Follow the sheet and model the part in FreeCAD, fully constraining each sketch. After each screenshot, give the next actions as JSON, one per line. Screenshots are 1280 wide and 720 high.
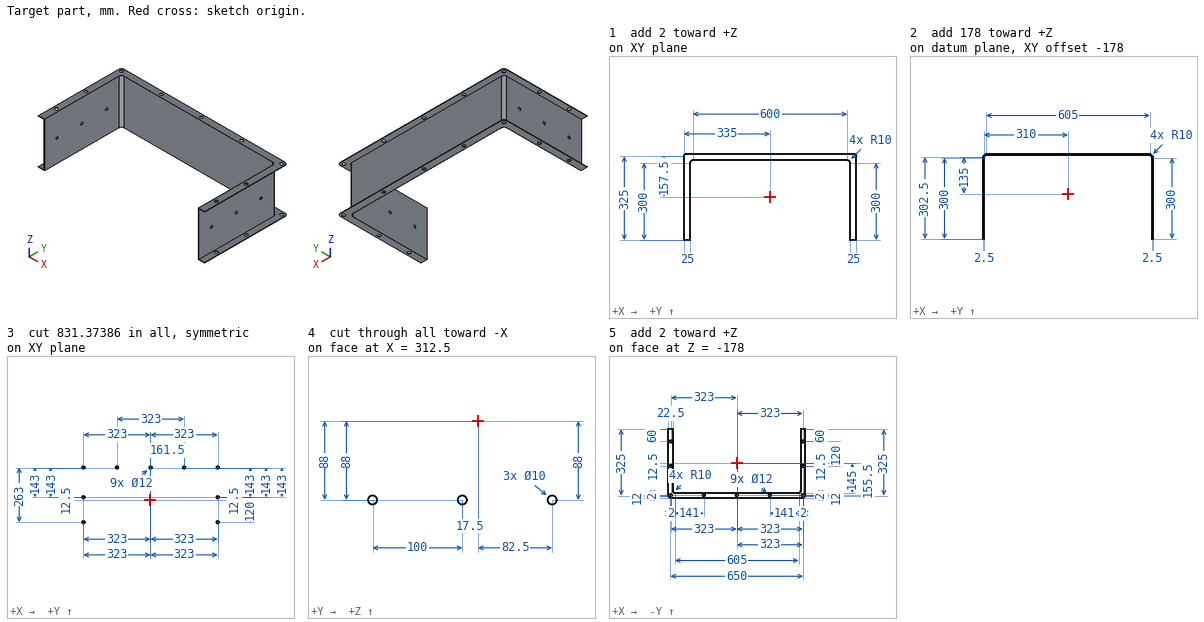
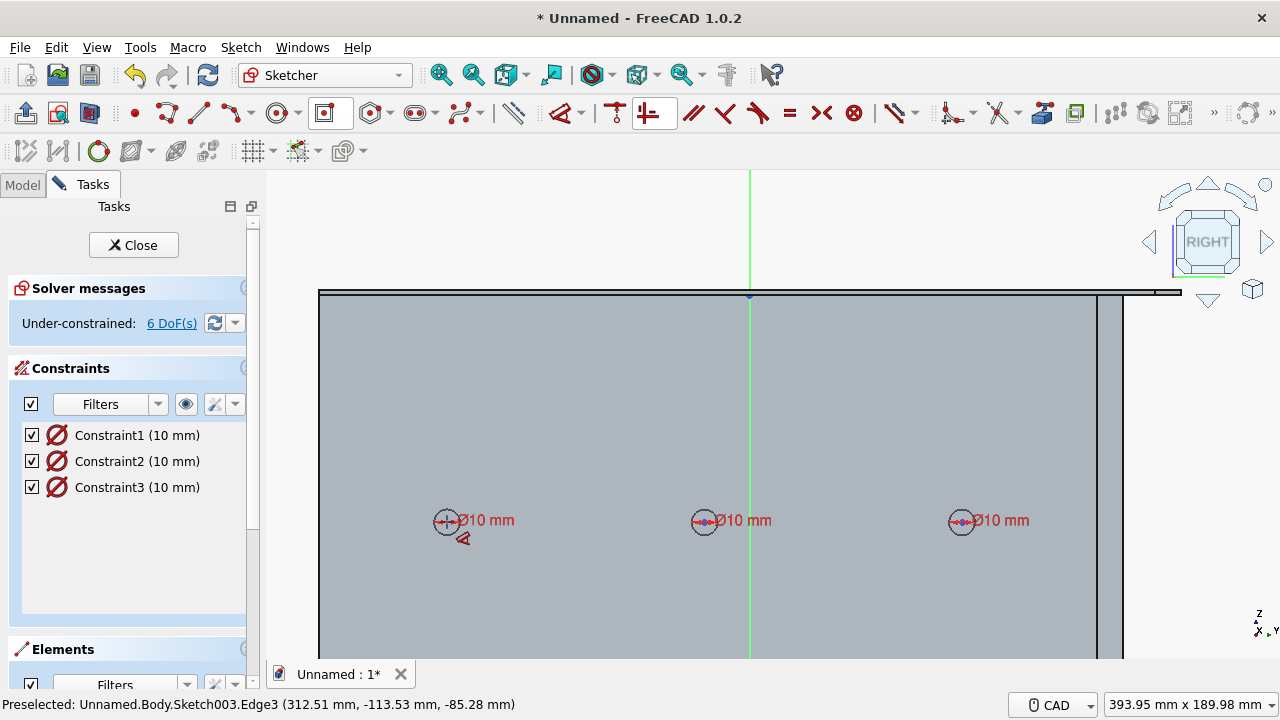
{"action": "left_click", "coordinate": [962, 522]}
{"action": "left_click", "coordinate": [996, 409]}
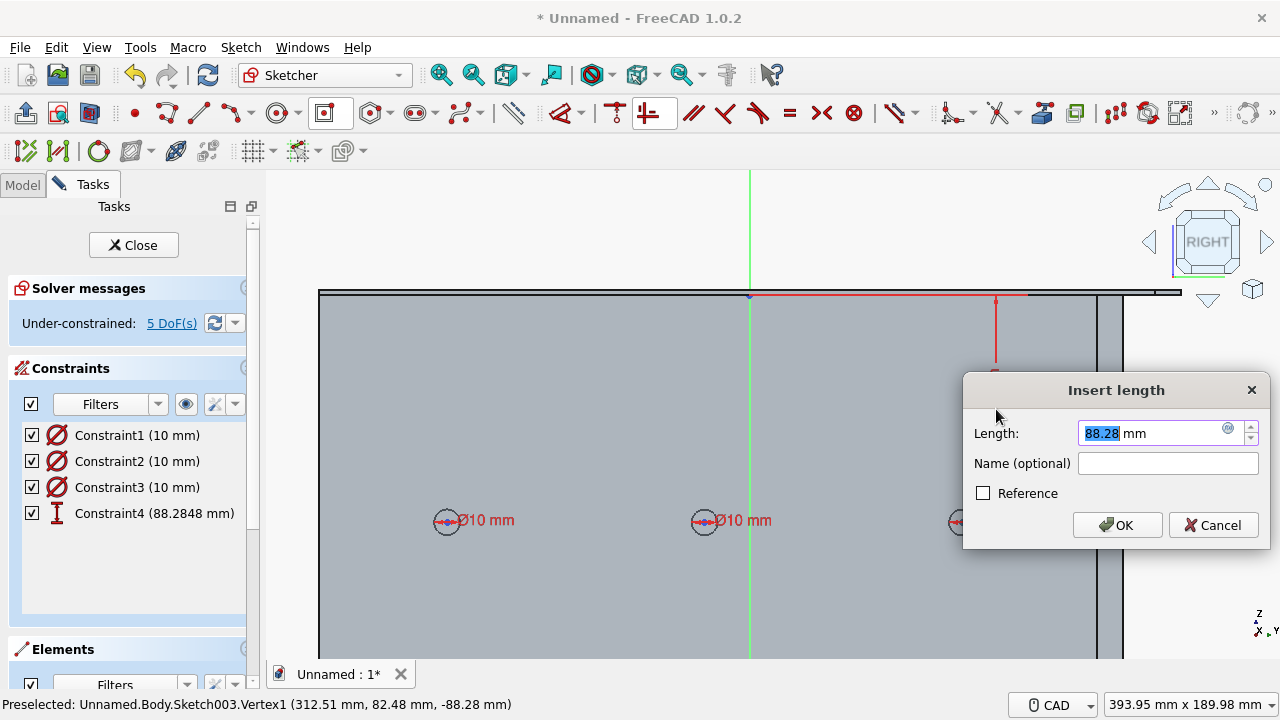
{"action": "type", "text": "88"}
{"action": "key", "text": "Return"}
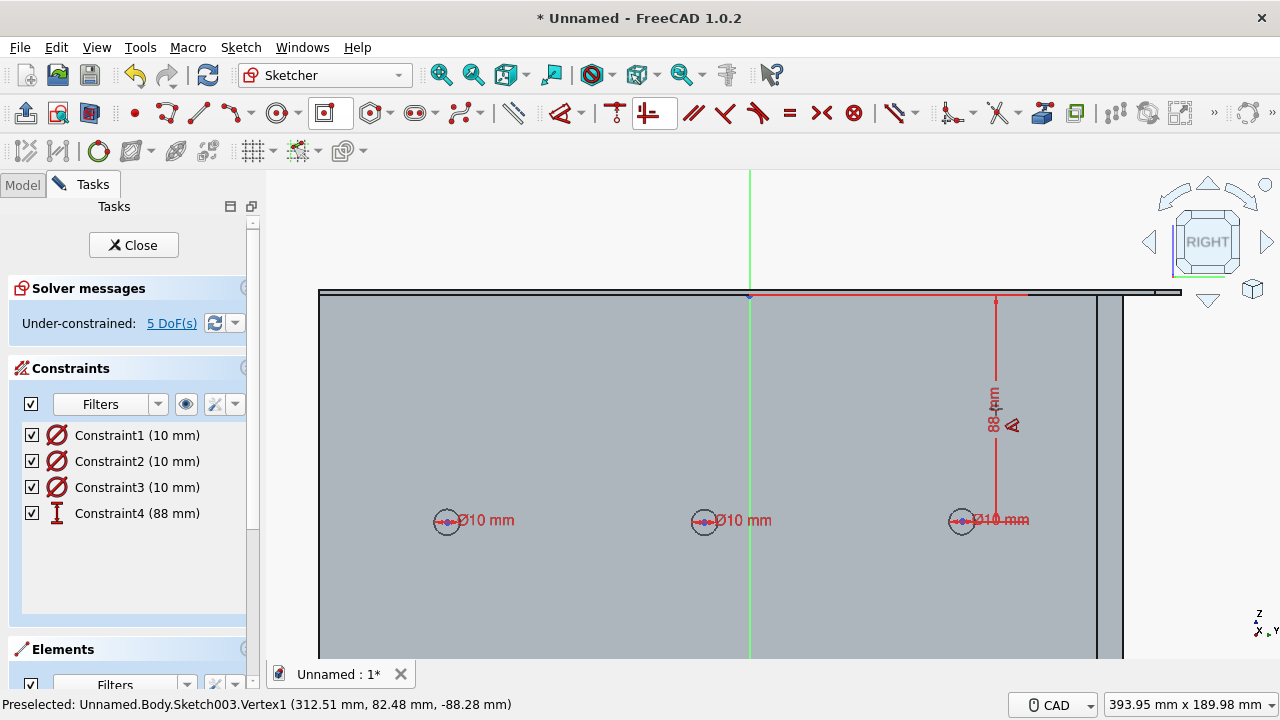
{"action": "left_click", "coordinate": [705, 522]}
{"action": "left_click", "coordinate": [784, 409]}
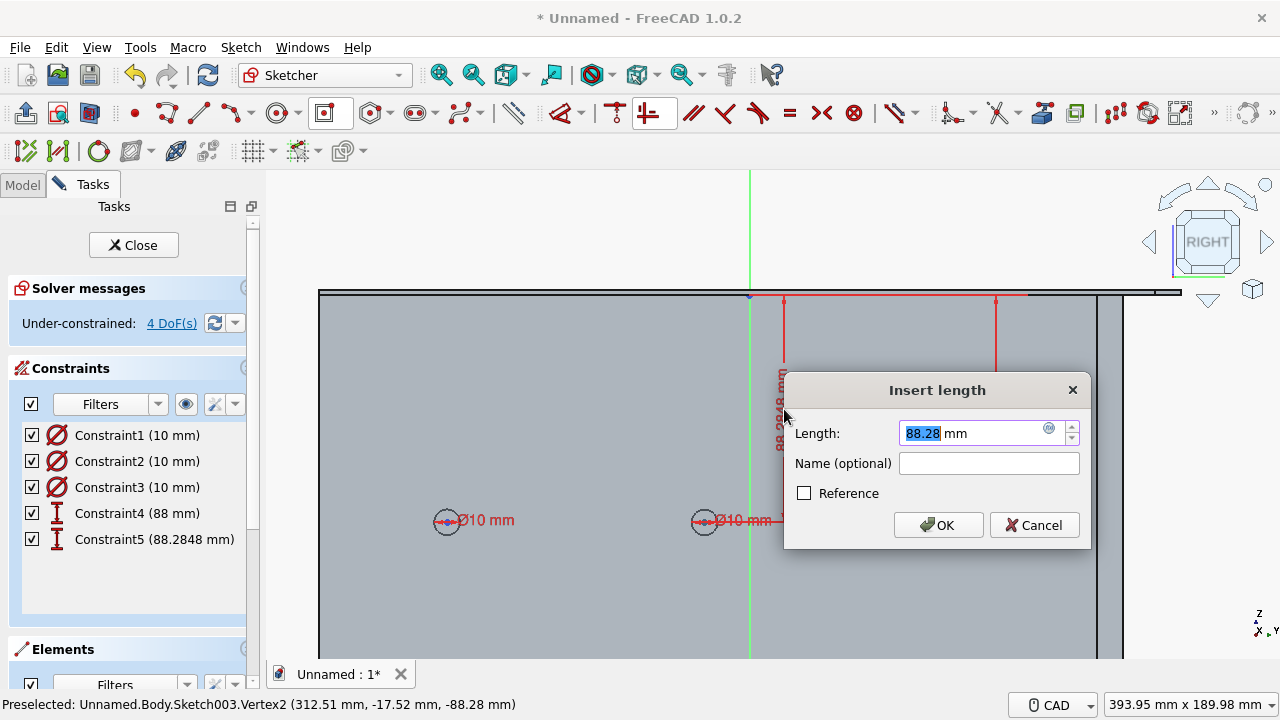
{"action": "type", "text": "88"}
{"action": "key", "text": "Return"}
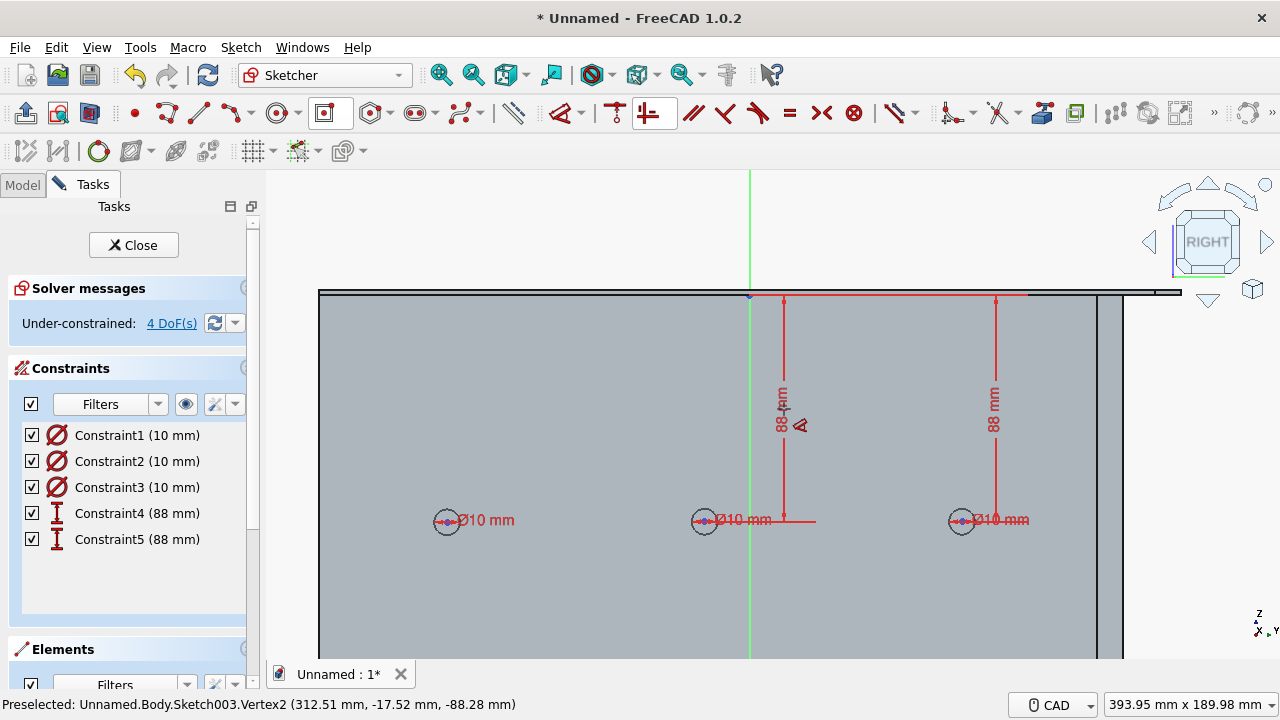
{"action": "left_click", "coordinate": [447, 522]}
{"action": "left_click", "coordinate": [413, 409]}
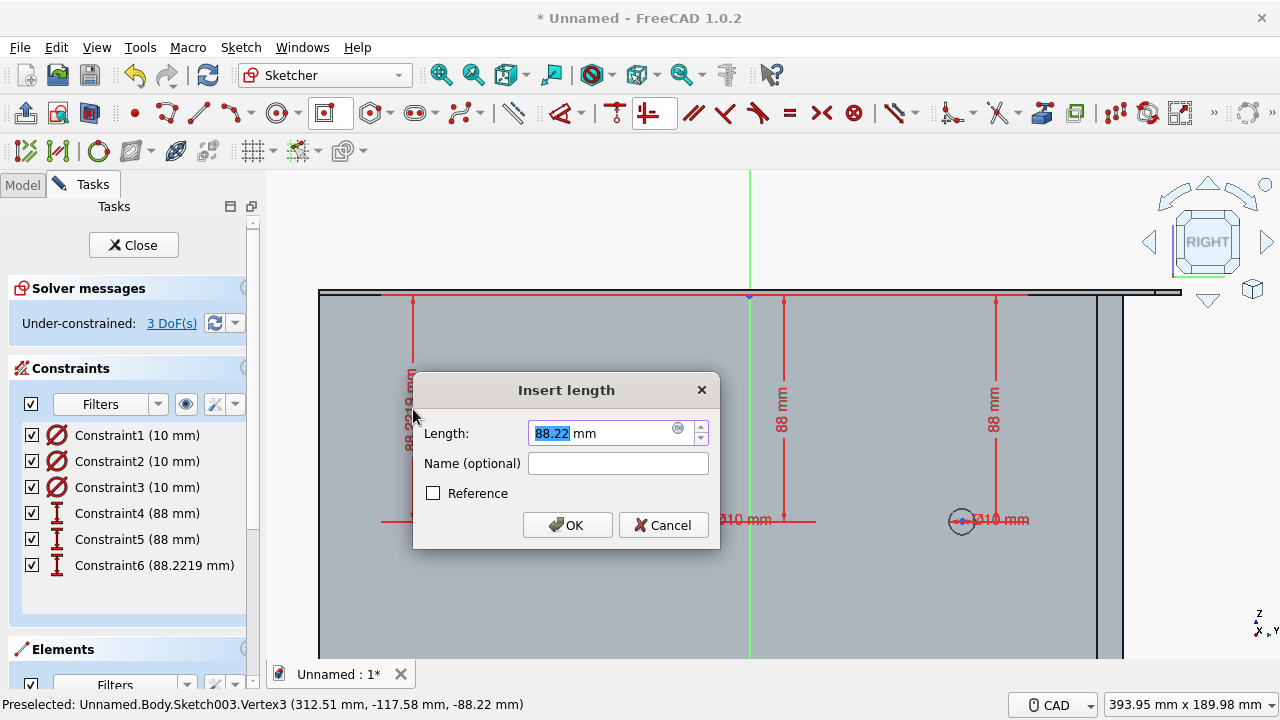
{"action": "type", "text": "88"}
{"action": "key", "text": "Return"}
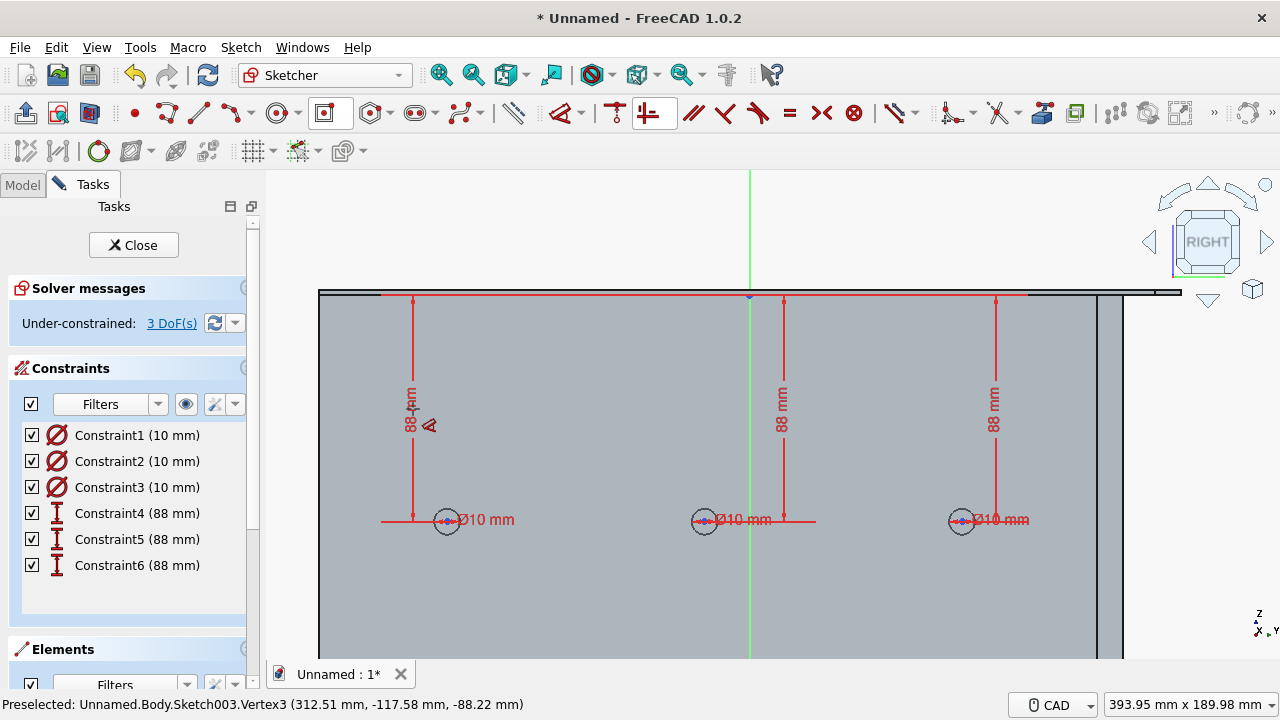
{"action": "left_click", "coordinate": [962, 522]}
{"action": "left_click", "coordinate": [856, 261]}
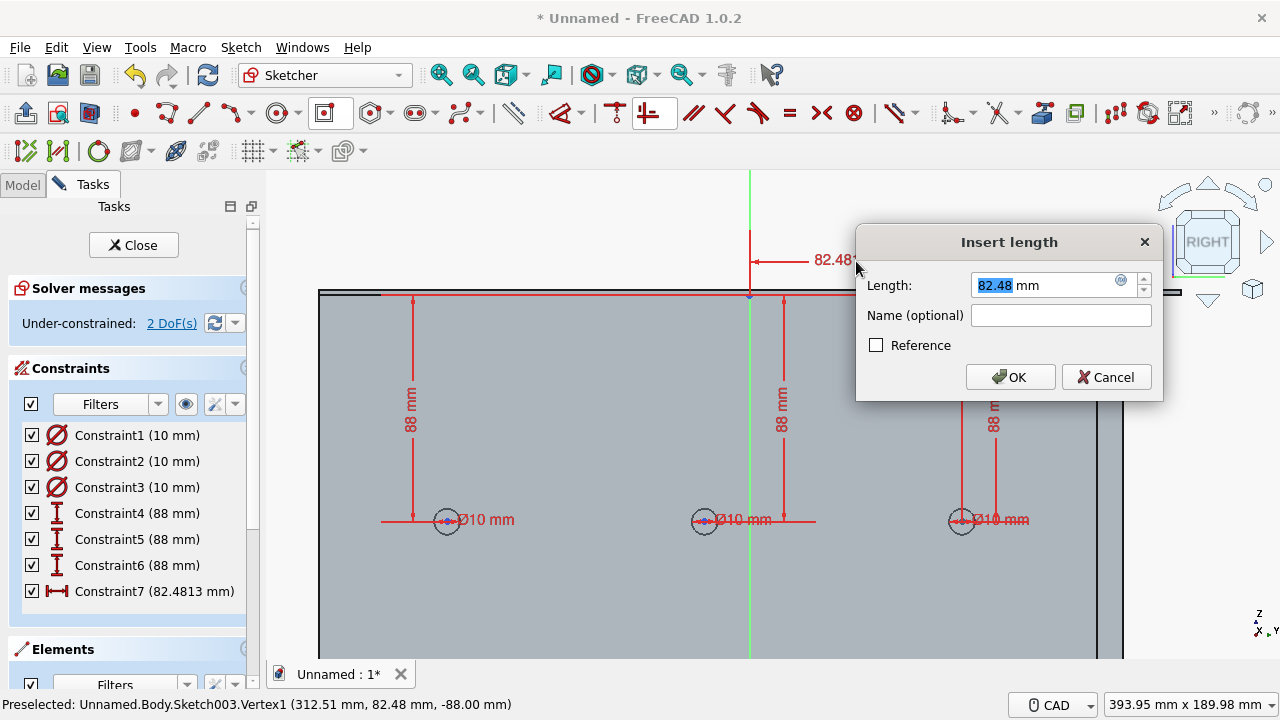
{"action": "type", "text": "82.5"}
{"action": "key", "text": "Return"}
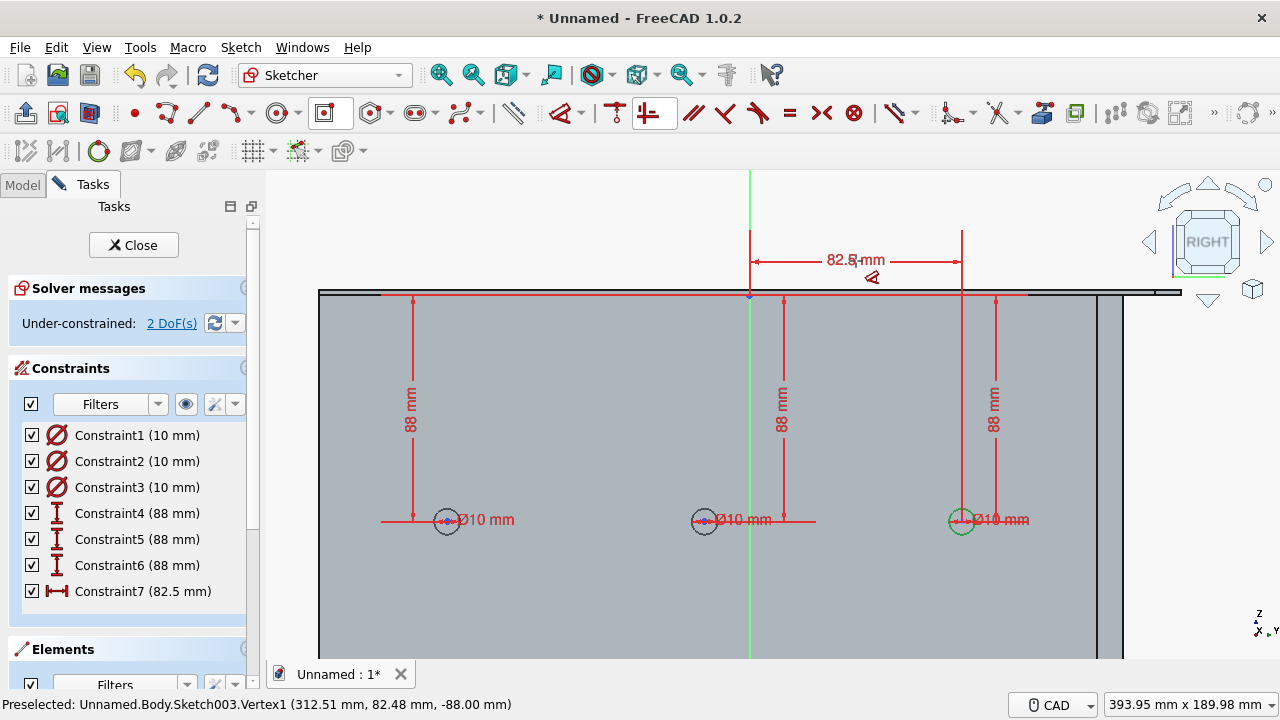
{"action": "left_click", "coordinate": [705, 522]}
{"action": "left_click", "coordinate": [727, 261]}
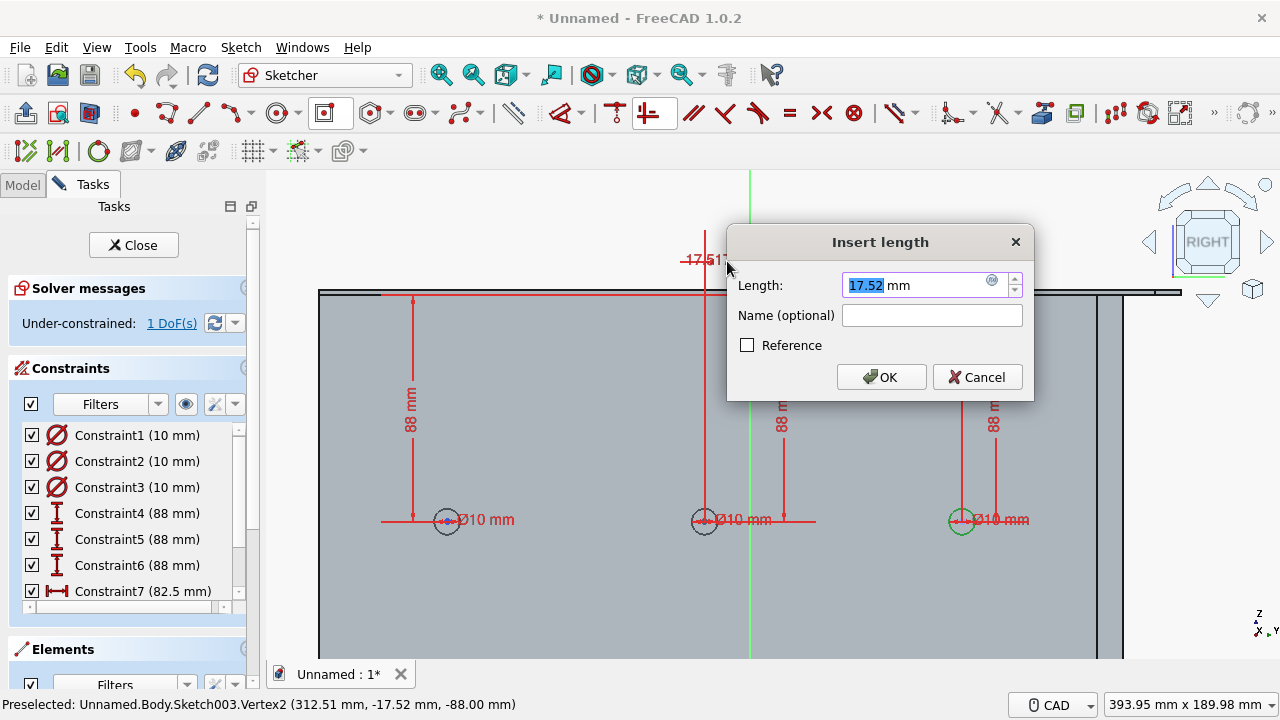
{"action": "type", "text": "17.5"}
{"action": "key", "text": "Return"}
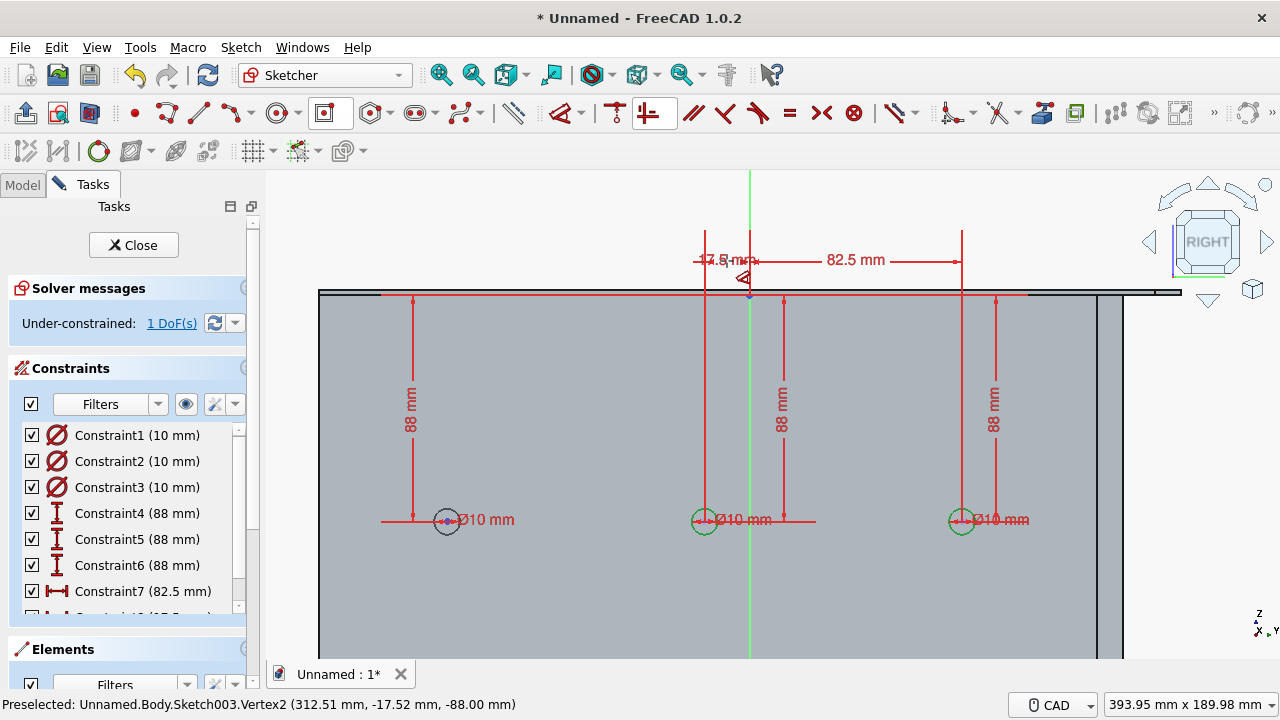
{"action": "left_click", "coordinate": [705, 522]}